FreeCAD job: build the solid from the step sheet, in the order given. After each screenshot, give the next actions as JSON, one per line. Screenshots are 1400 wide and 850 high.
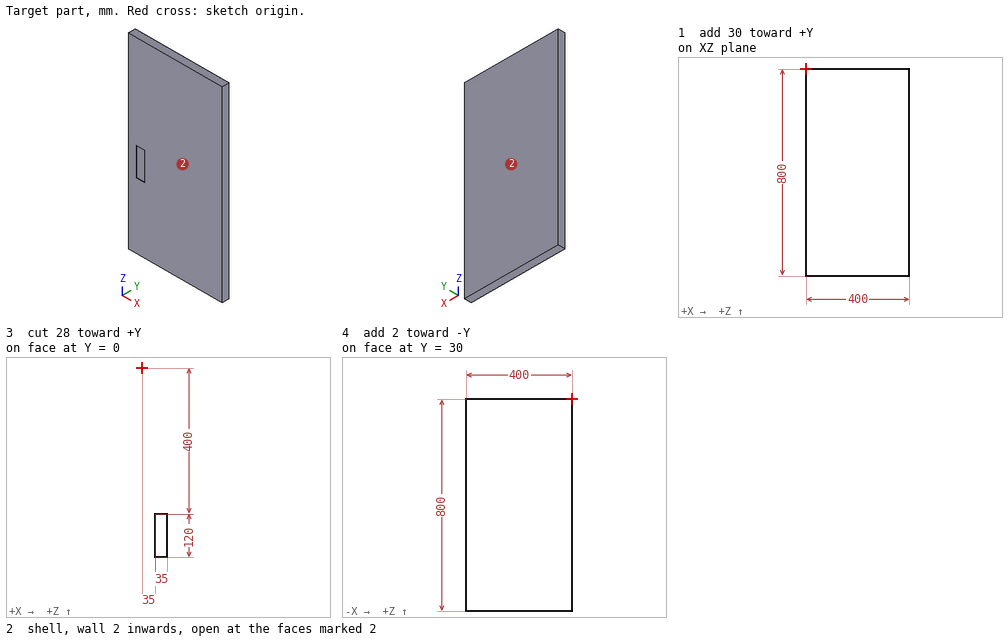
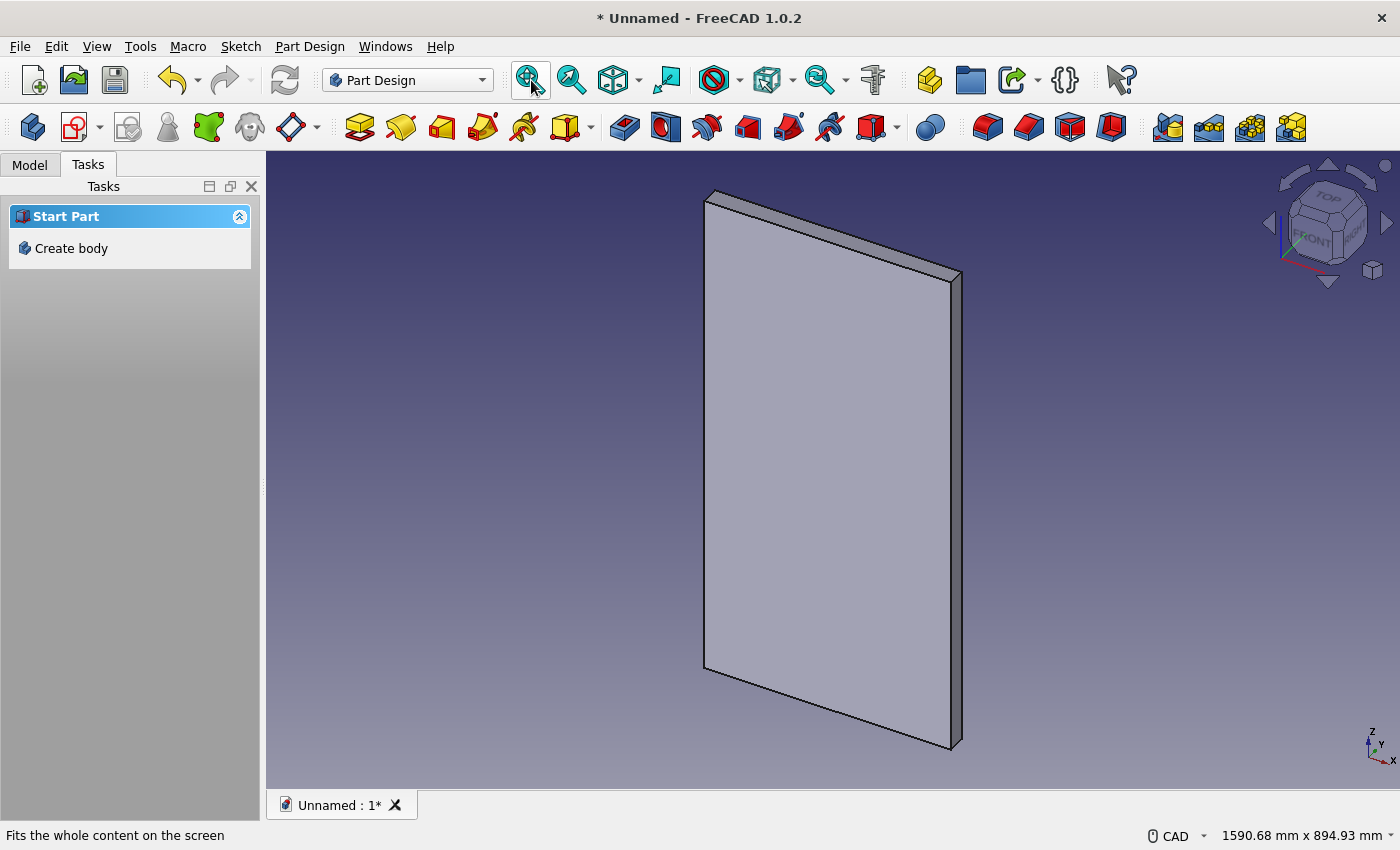
{"action": "key", "text": "0"}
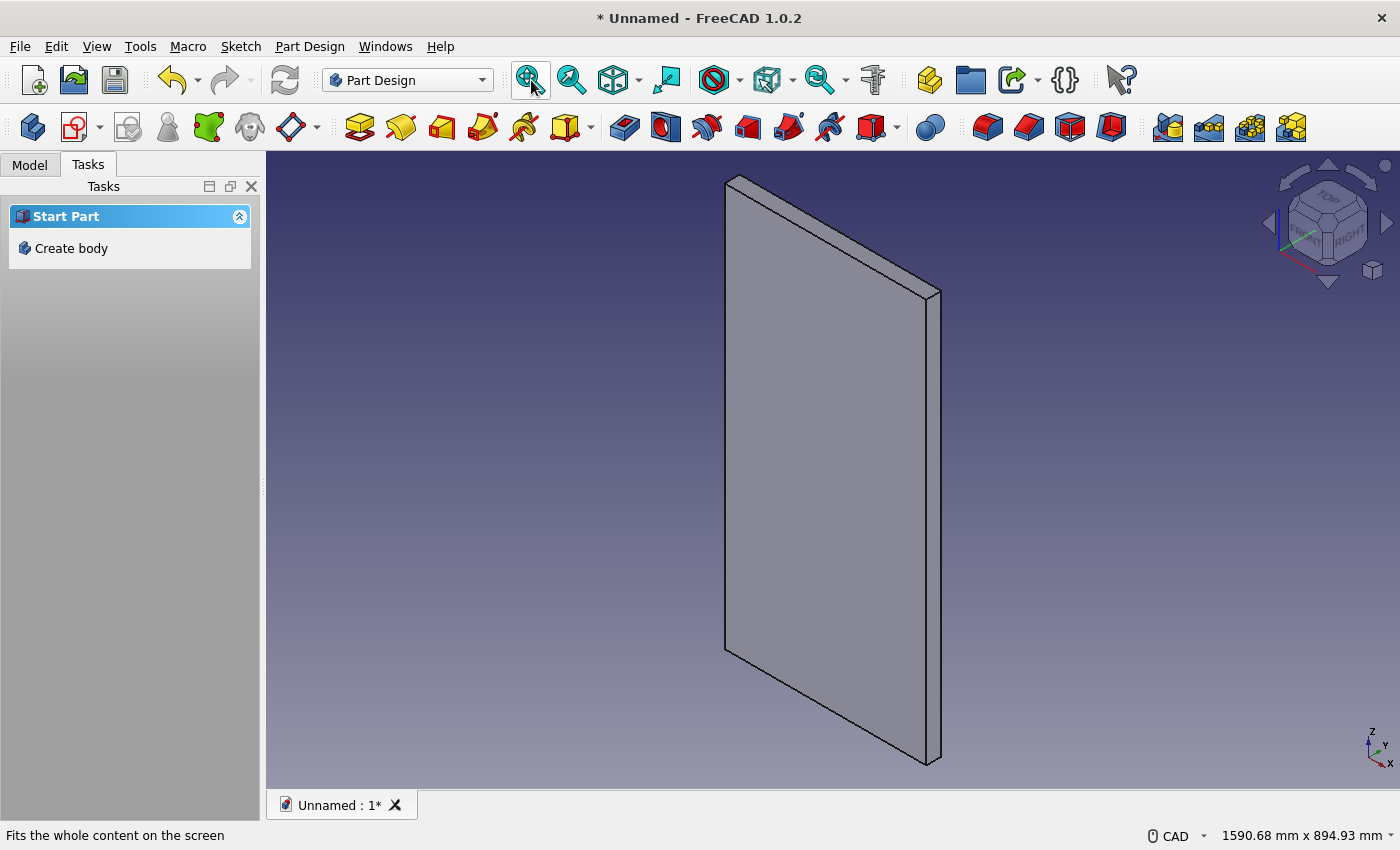
{"action": "key", "text": "2"}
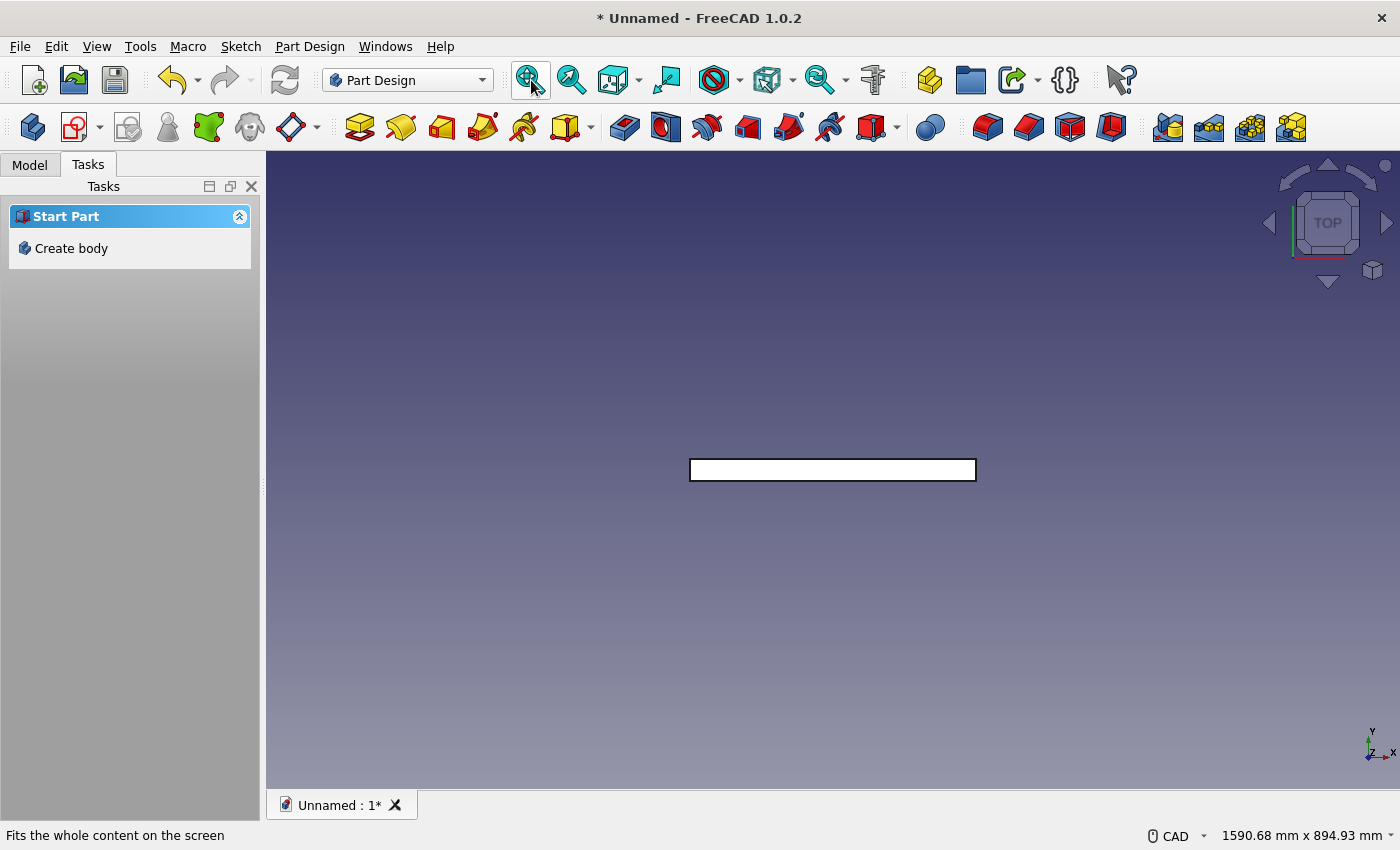
{"action": "left_click", "coordinate": [531, 80]}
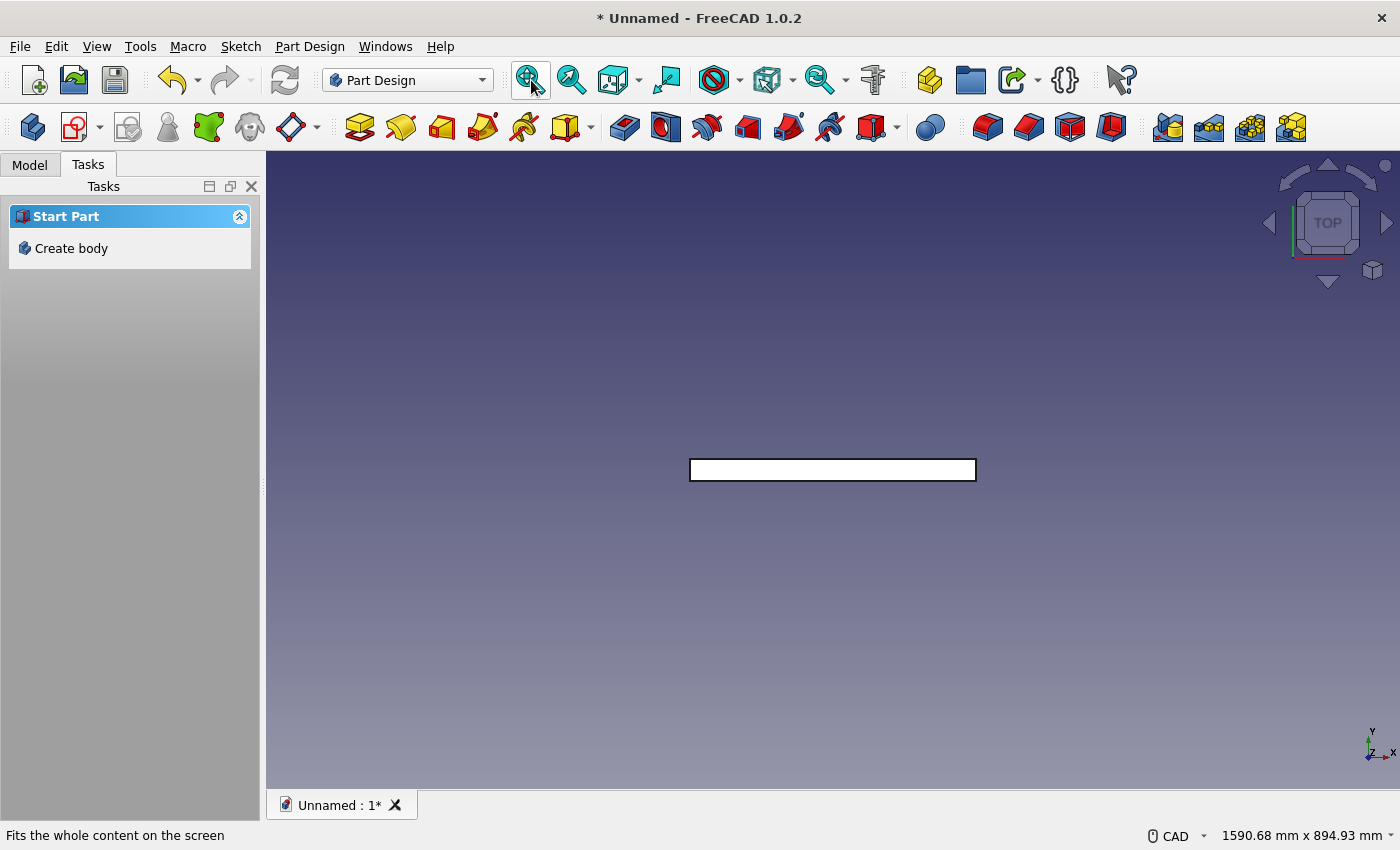
{"action": "key", "text": "1"}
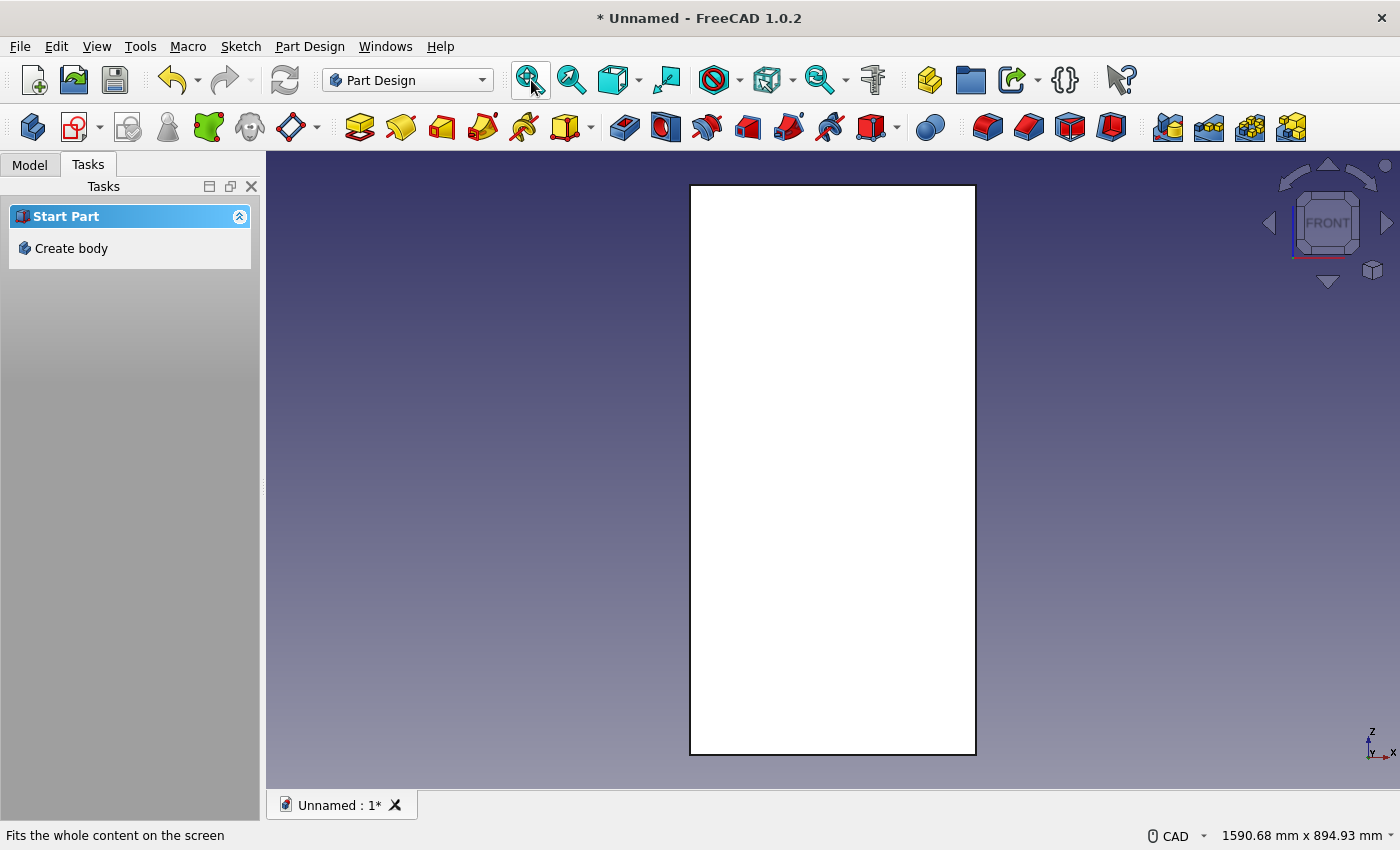
{"action": "key", "text": "3"}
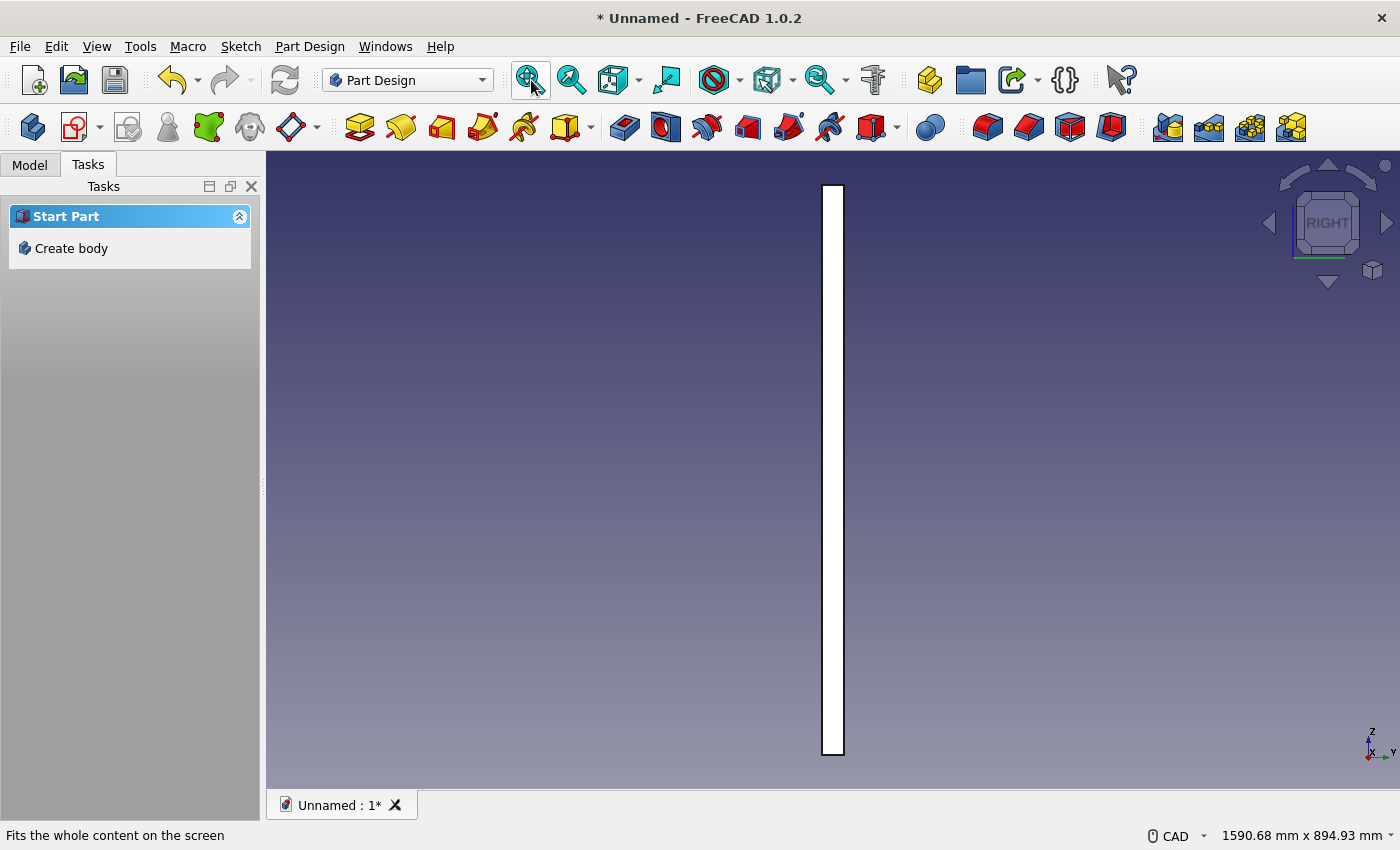
{"action": "key", "text": "5"}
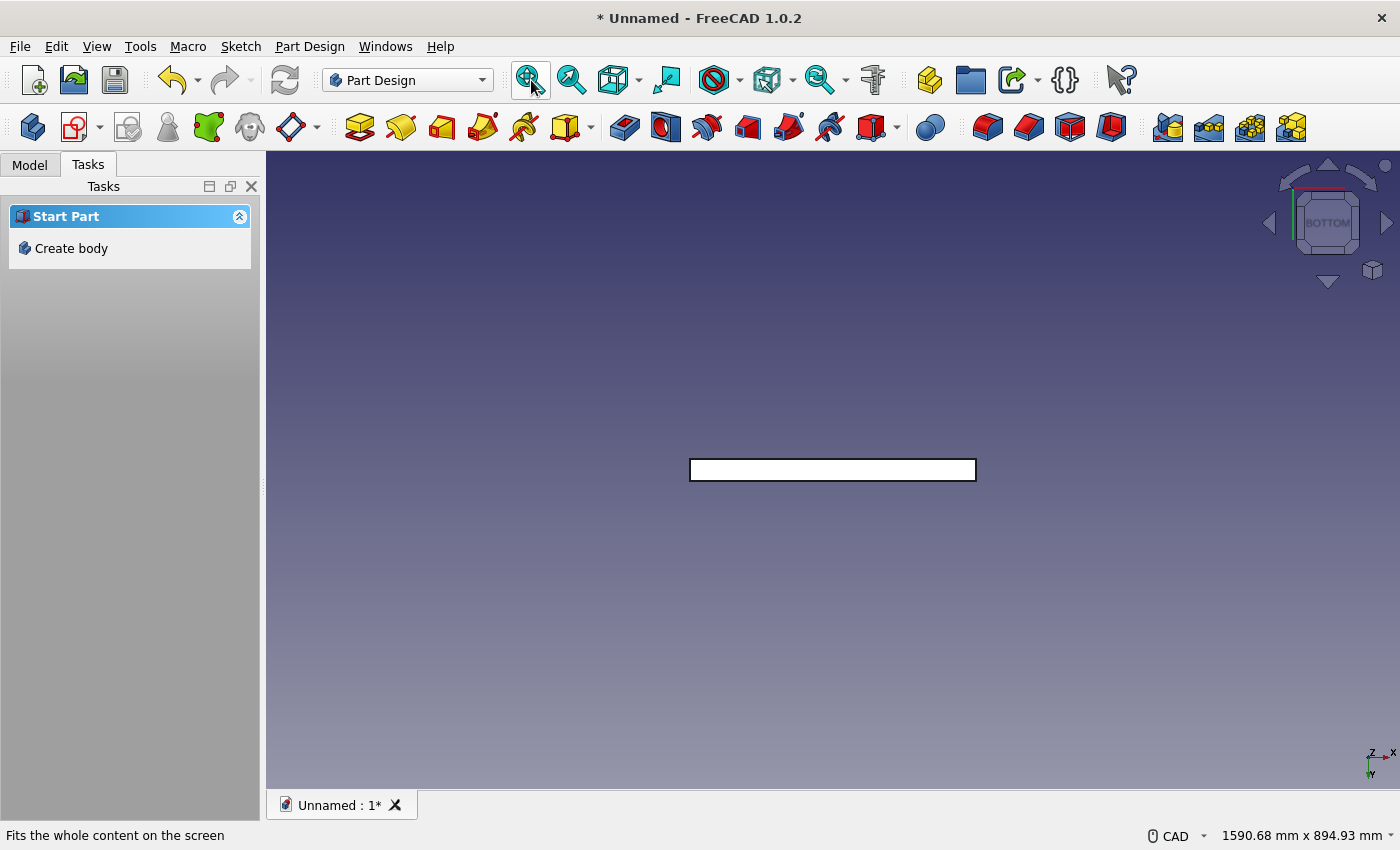
{"action": "left_click", "coordinate": [531, 80]}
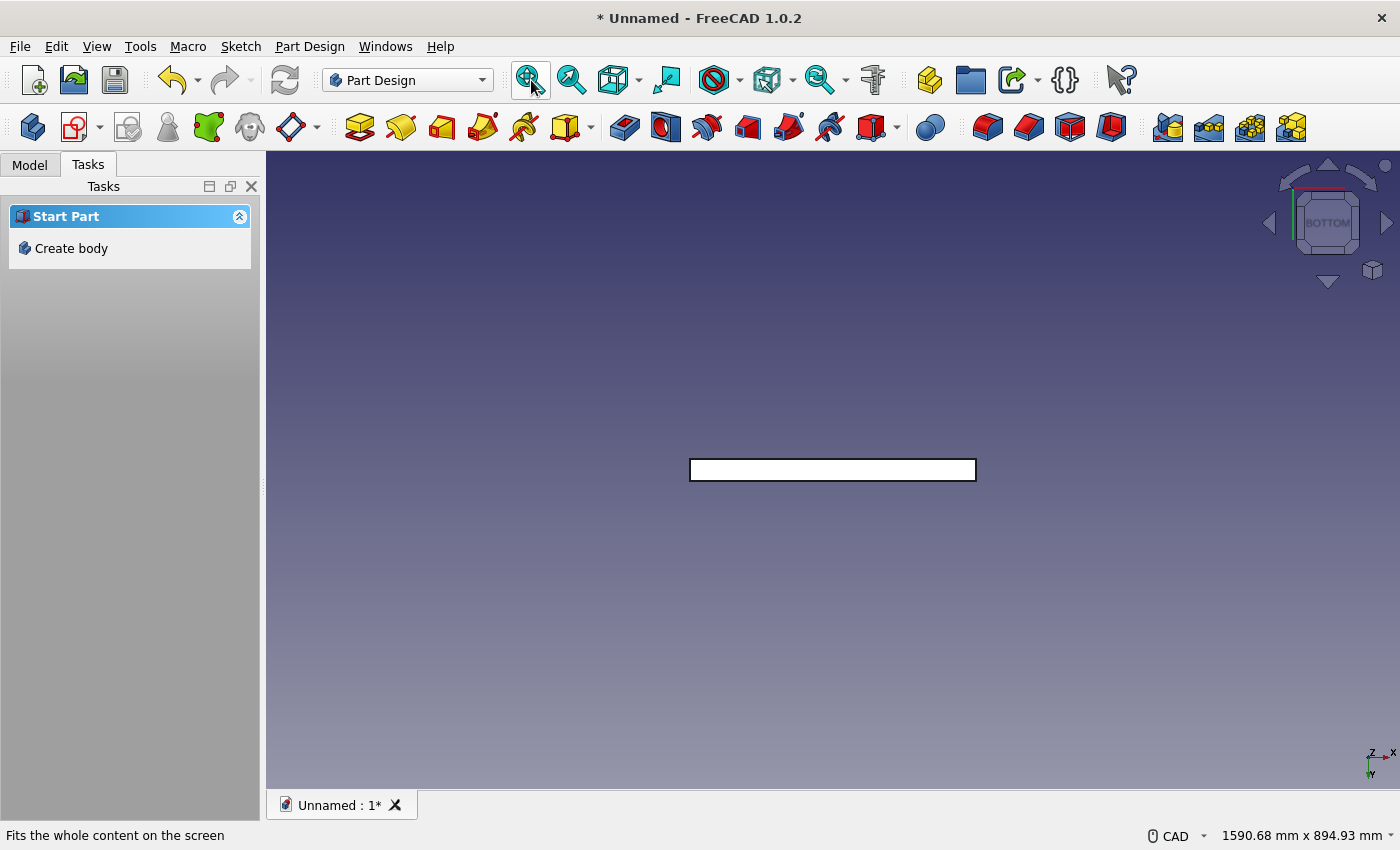
{"action": "key", "text": "4"}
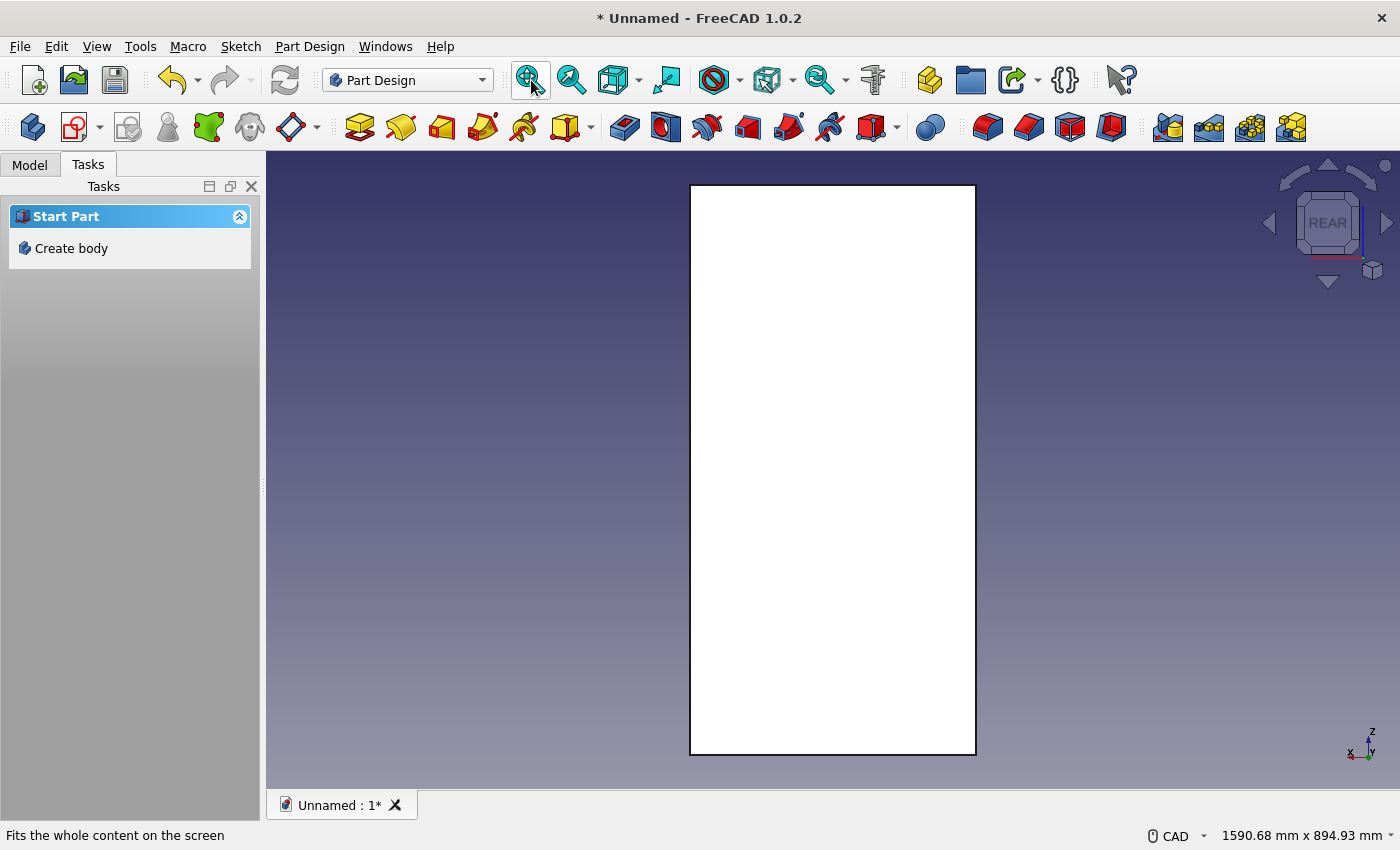
{"action": "left_click", "coordinate": [833, 388]}